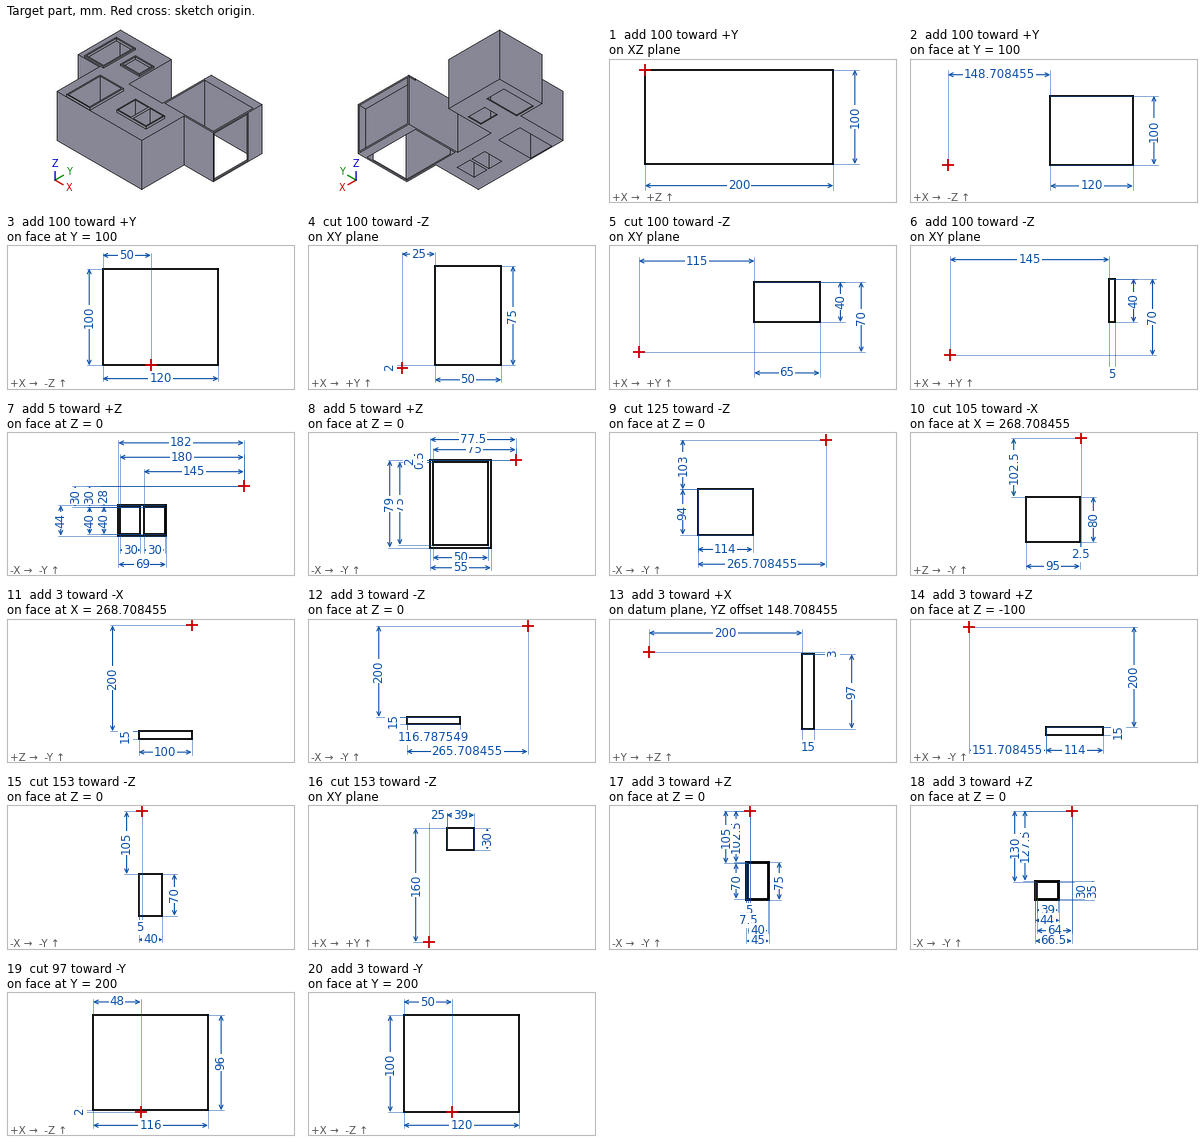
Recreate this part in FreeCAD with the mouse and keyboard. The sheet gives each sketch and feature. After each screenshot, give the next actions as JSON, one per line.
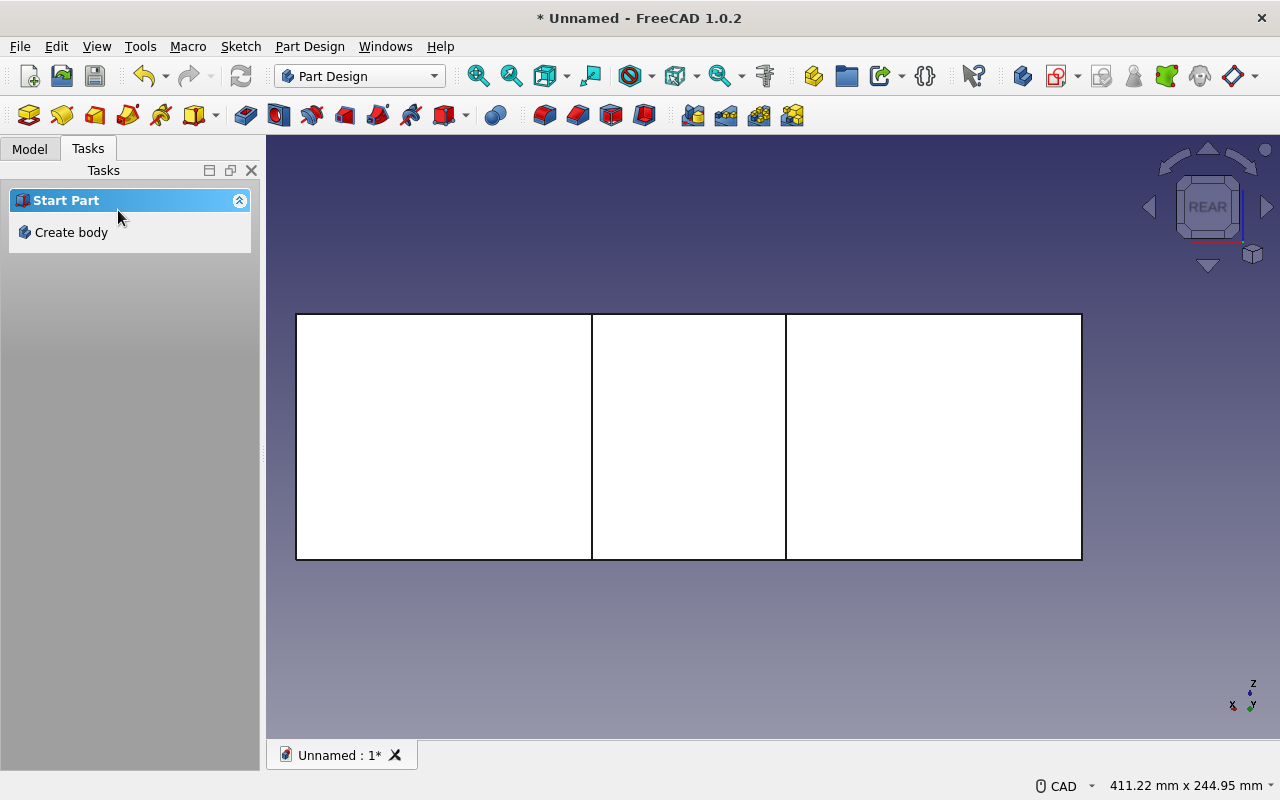
{"action": "left_click", "coordinate": [1056, 76]}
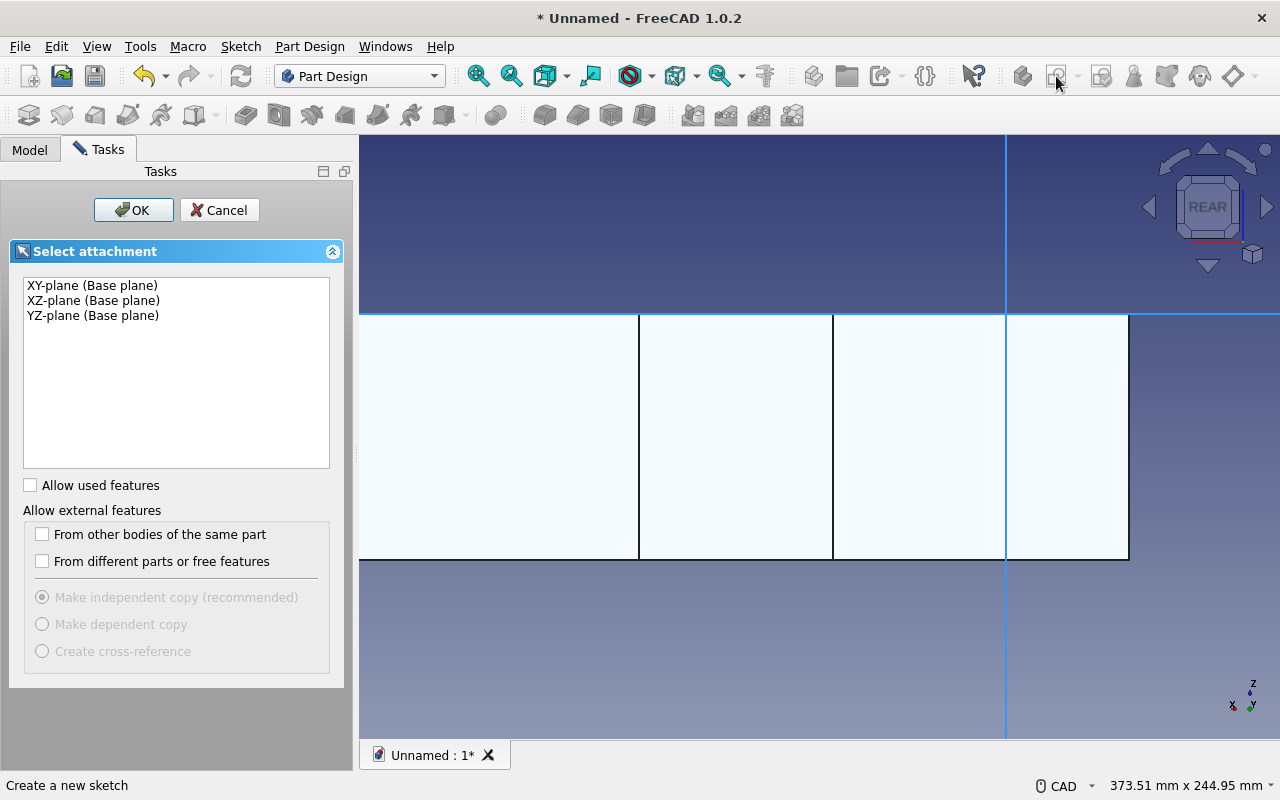
{"action": "left_click", "coordinate": [84, 286]}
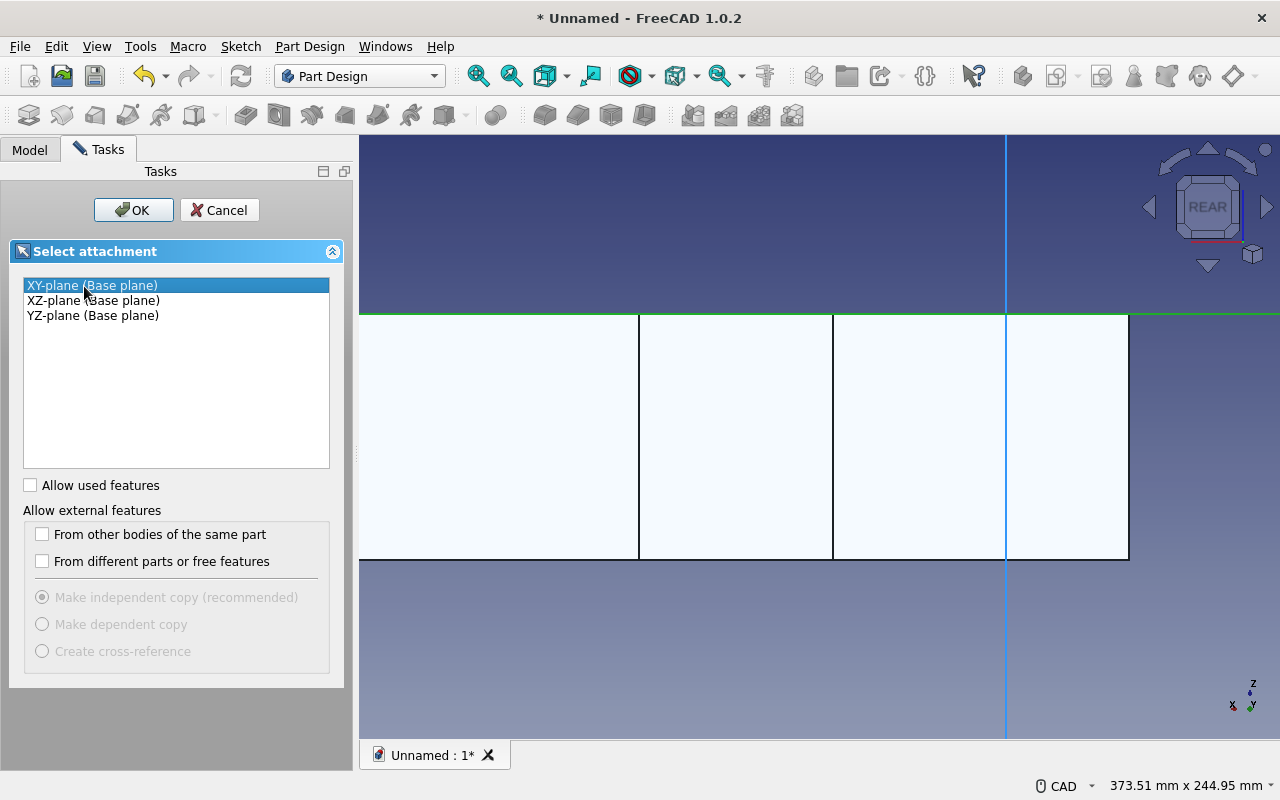
{"action": "left_click", "coordinate": [134, 210]}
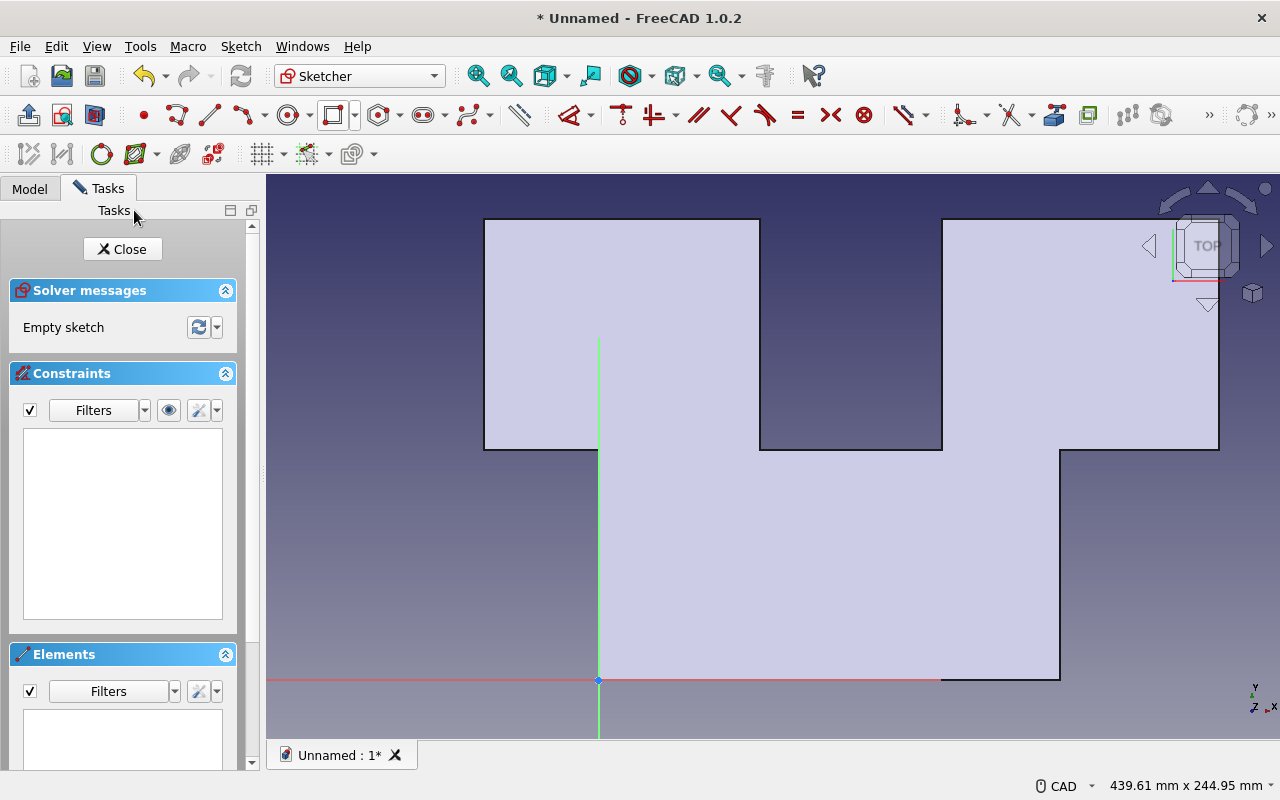
{"action": "scroll", "coordinate": [670, 702], "scroll_direction": "up", "scroll_amount": 4}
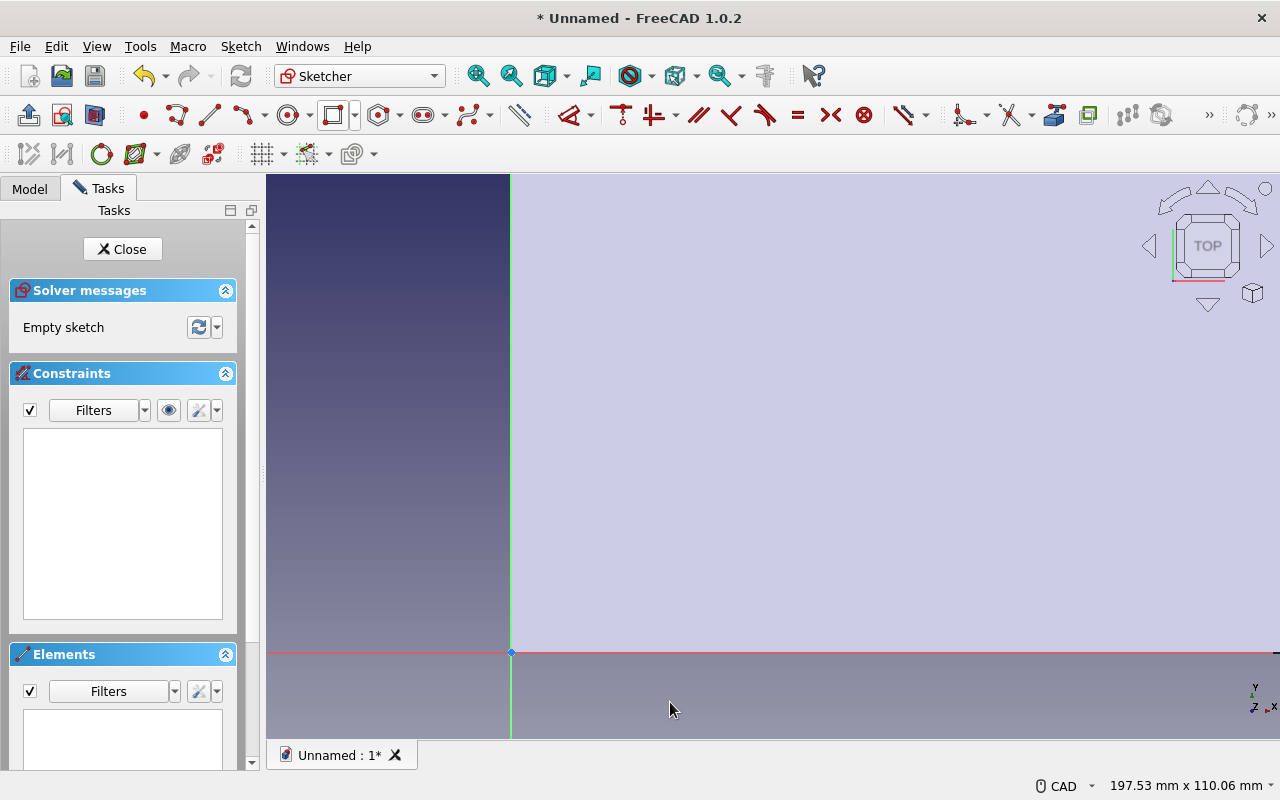
{"action": "left_click", "coordinate": [332, 116]}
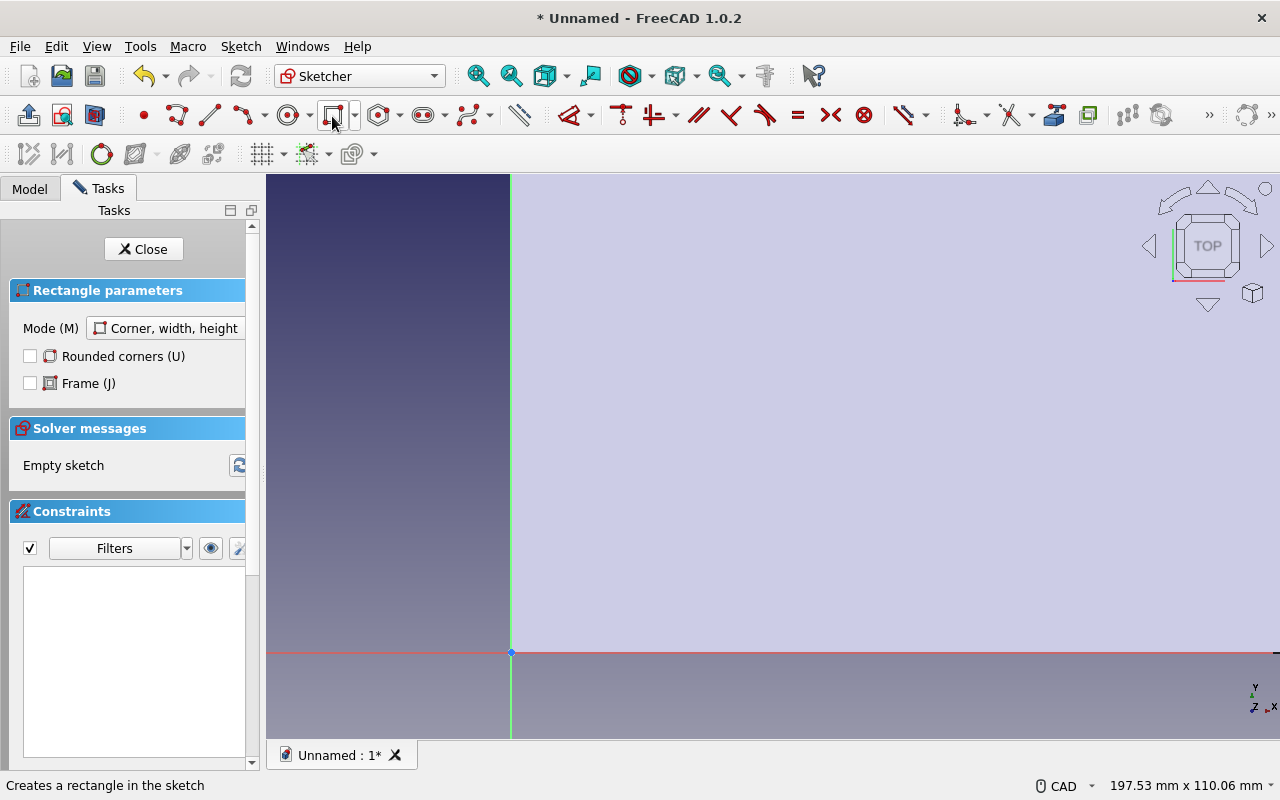
{"action": "left_click", "coordinate": [640, 257]}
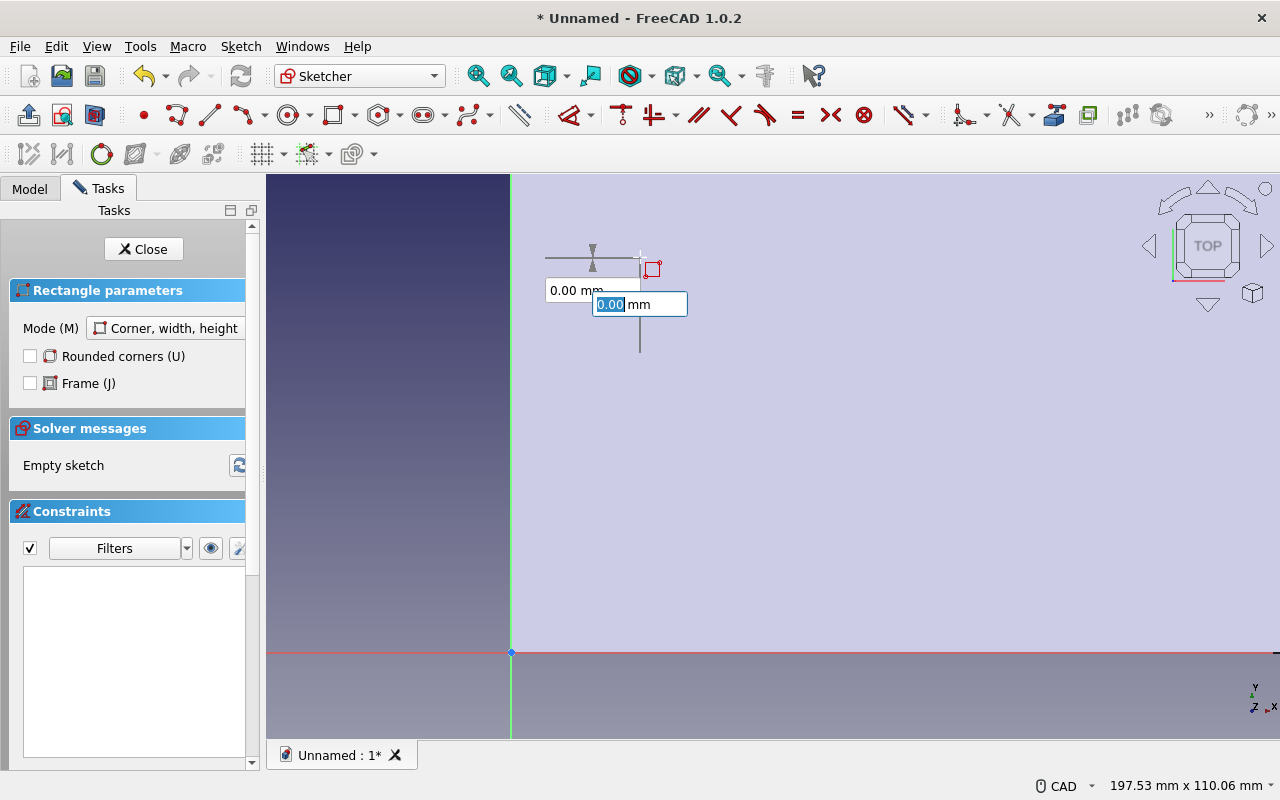
{"action": "scroll", "coordinate": [896, 642], "scroll_direction": "up", "scroll_amount": 3}
{"action": "mouse_move", "coordinate": [896, 642]}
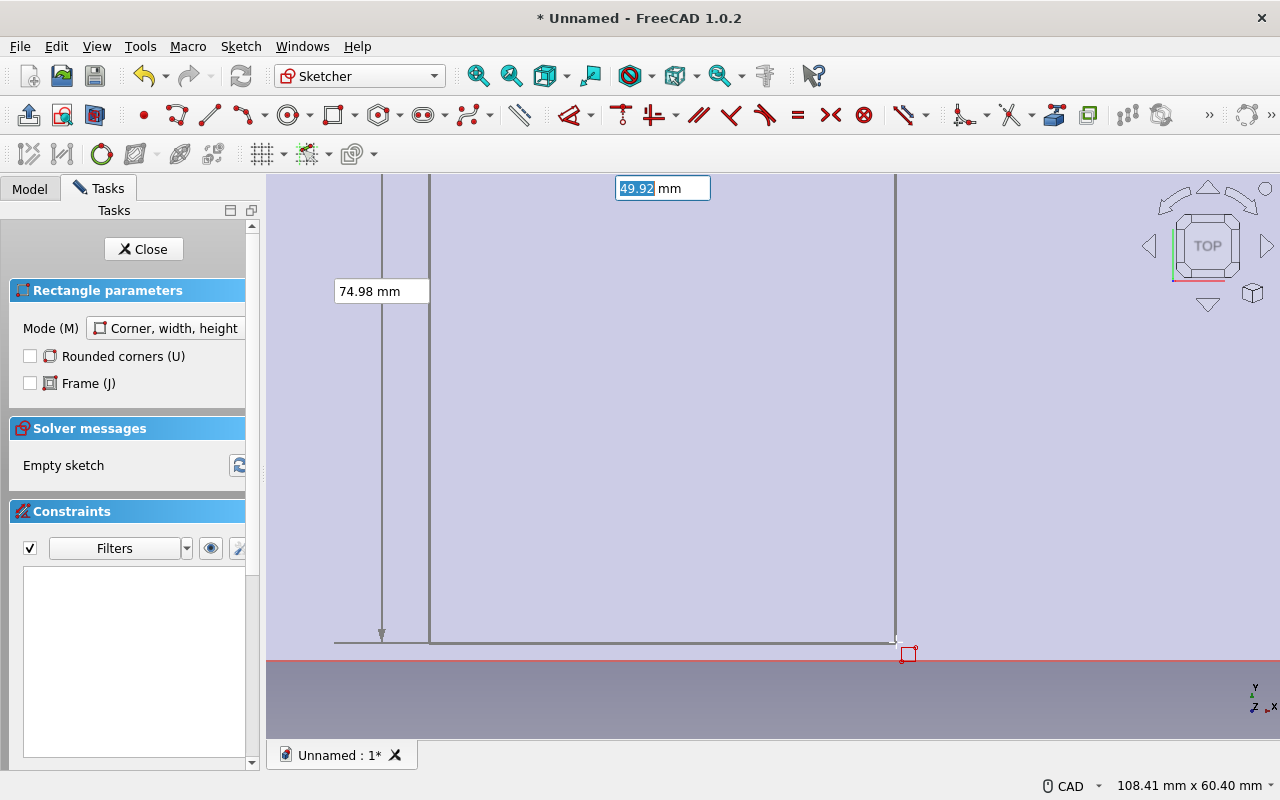
{"action": "type", "text": "50"}
{"action": "key", "text": "Tab"}
{"action": "type", "text": "75"}
{"action": "key", "text": "Return"}
{"action": "key", "text": "Escape"}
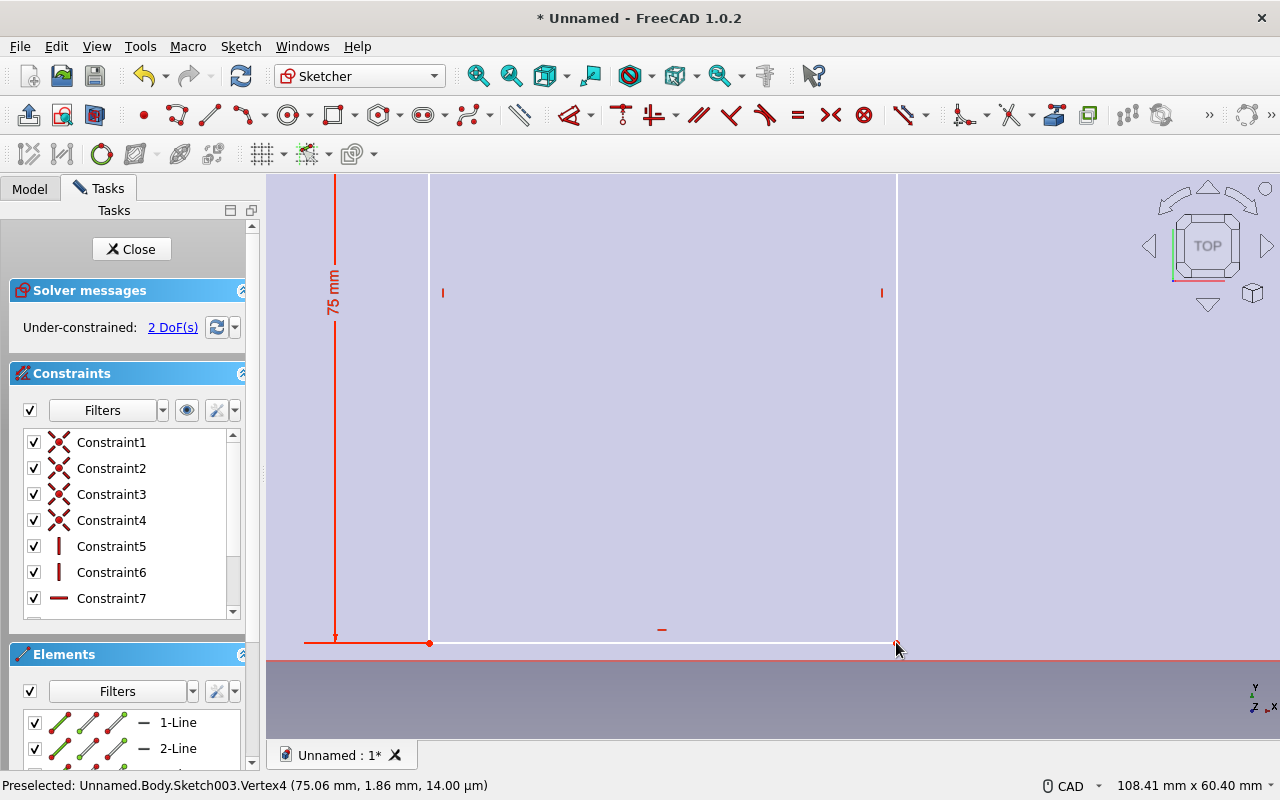
{"action": "left_click", "coordinate": [568, 116]}